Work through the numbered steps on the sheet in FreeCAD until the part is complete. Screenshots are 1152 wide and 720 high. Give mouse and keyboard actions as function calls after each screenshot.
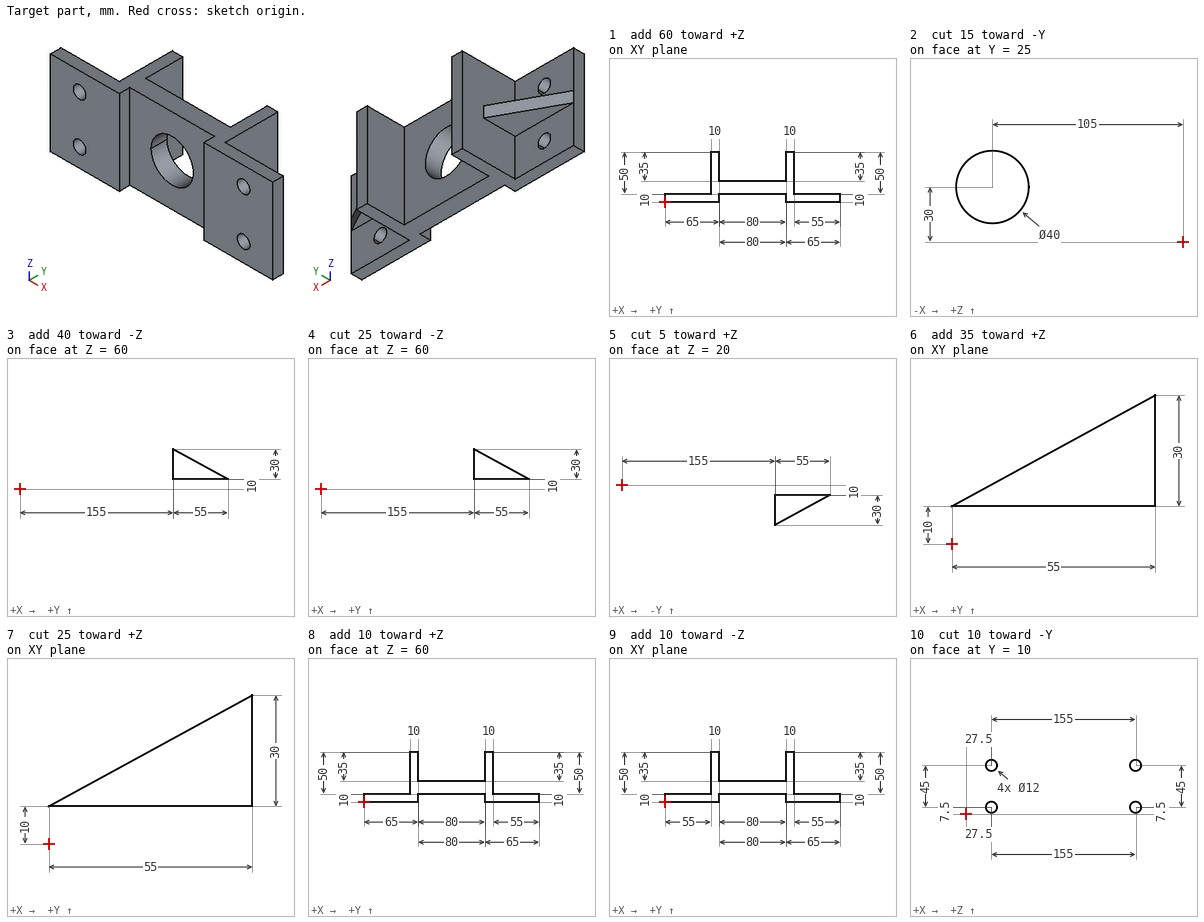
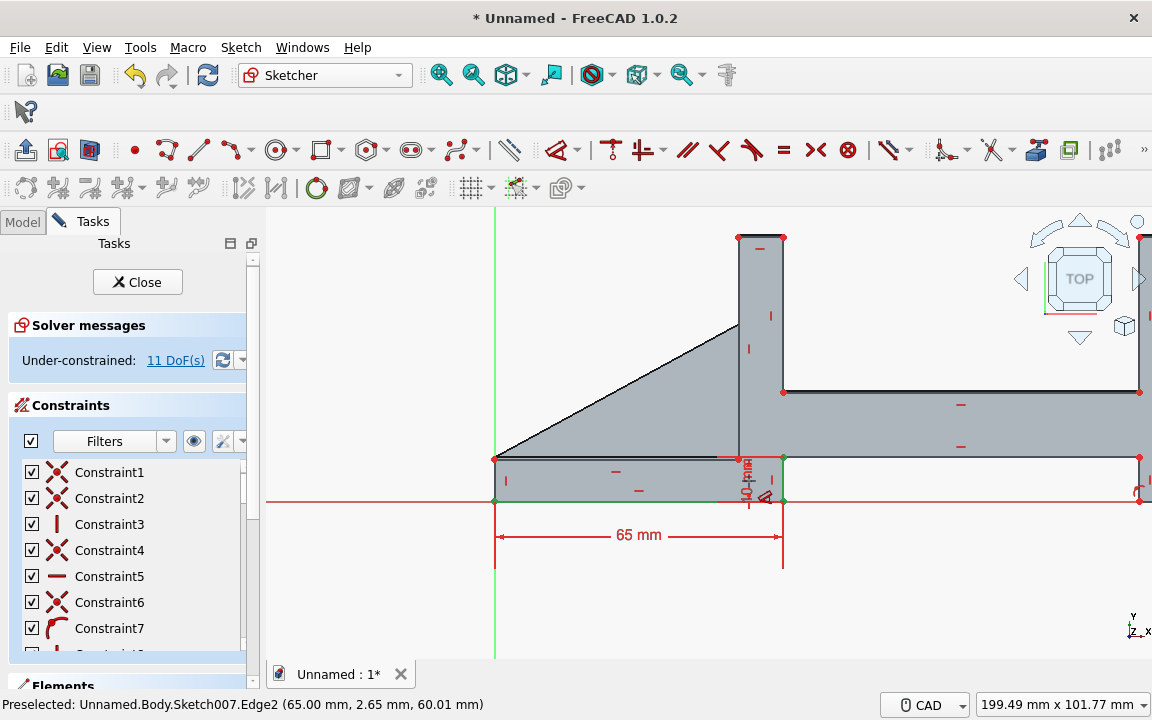
click(890, 457)
click(885, 423)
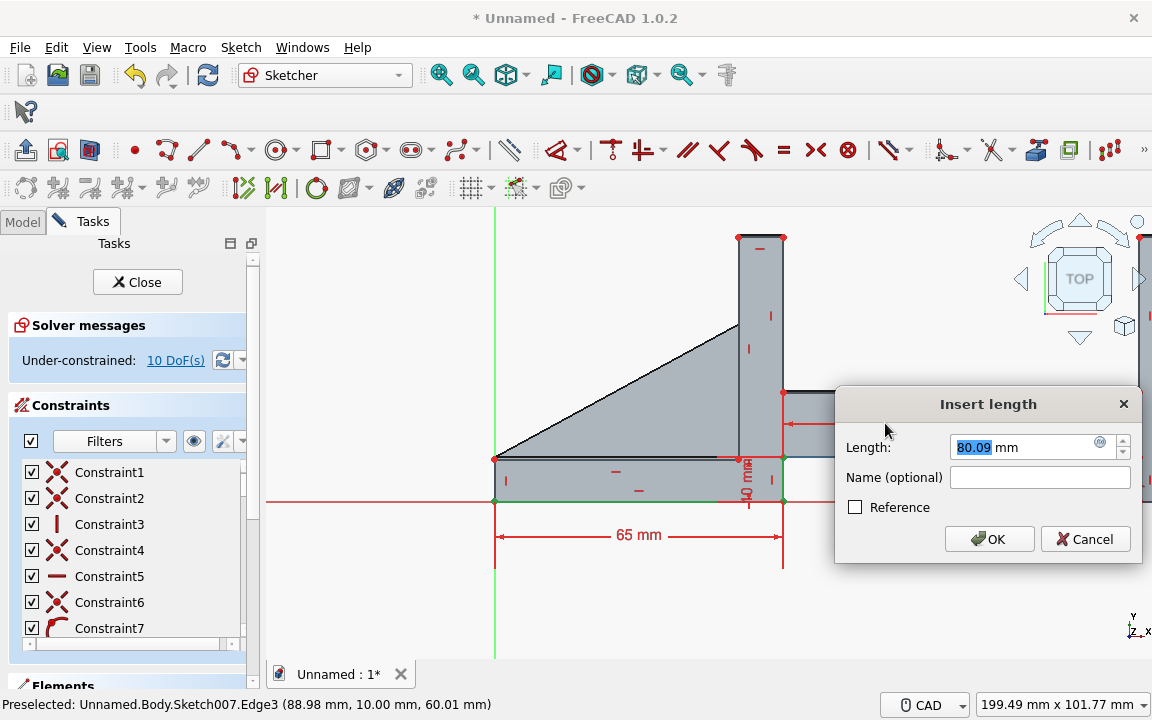
text(80)
key(Return)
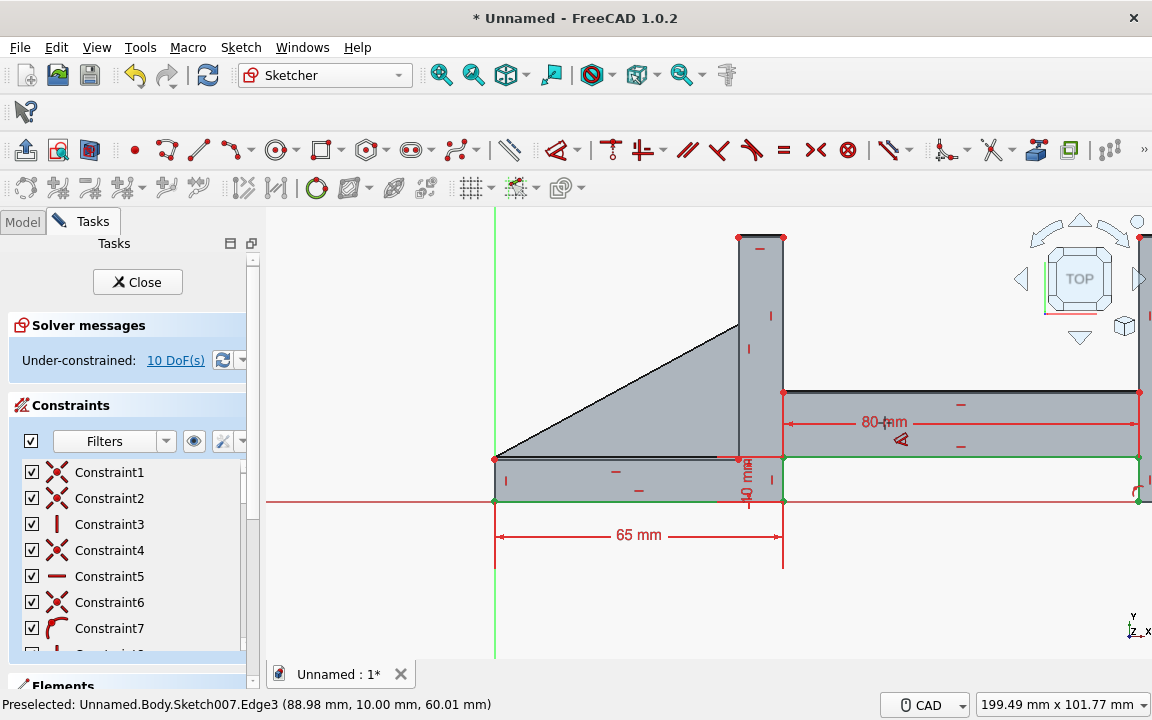
scroll(294, 511, down, 3)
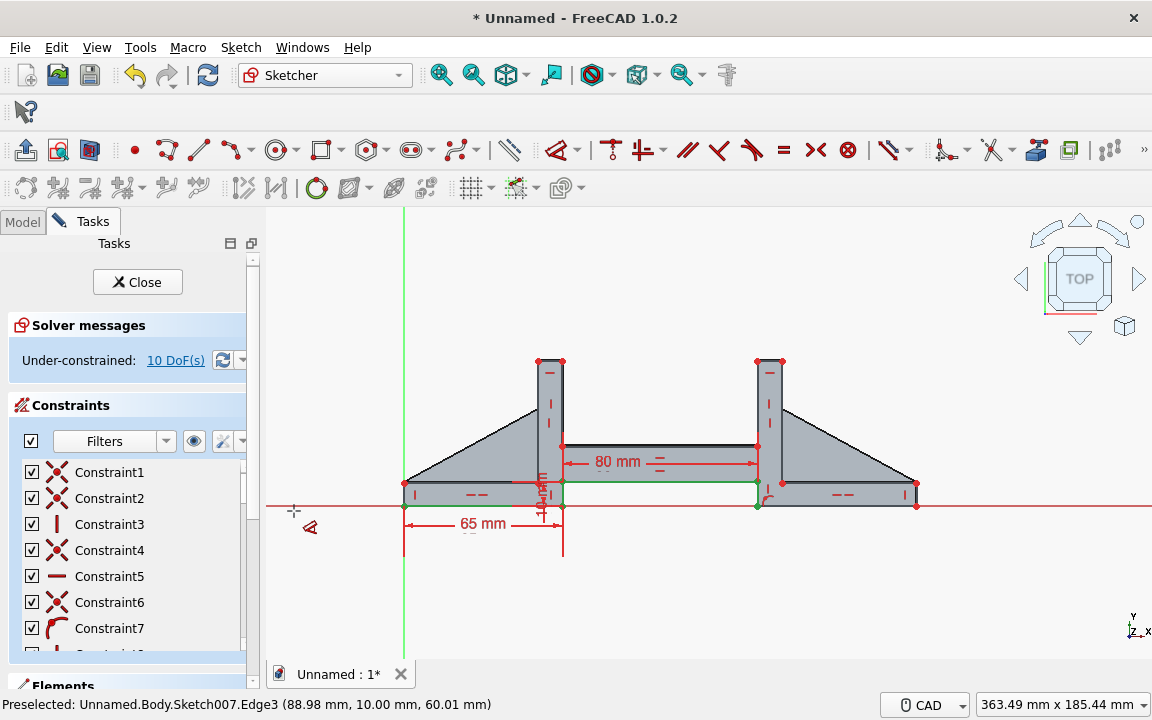
click(805, 506)
click(837, 540)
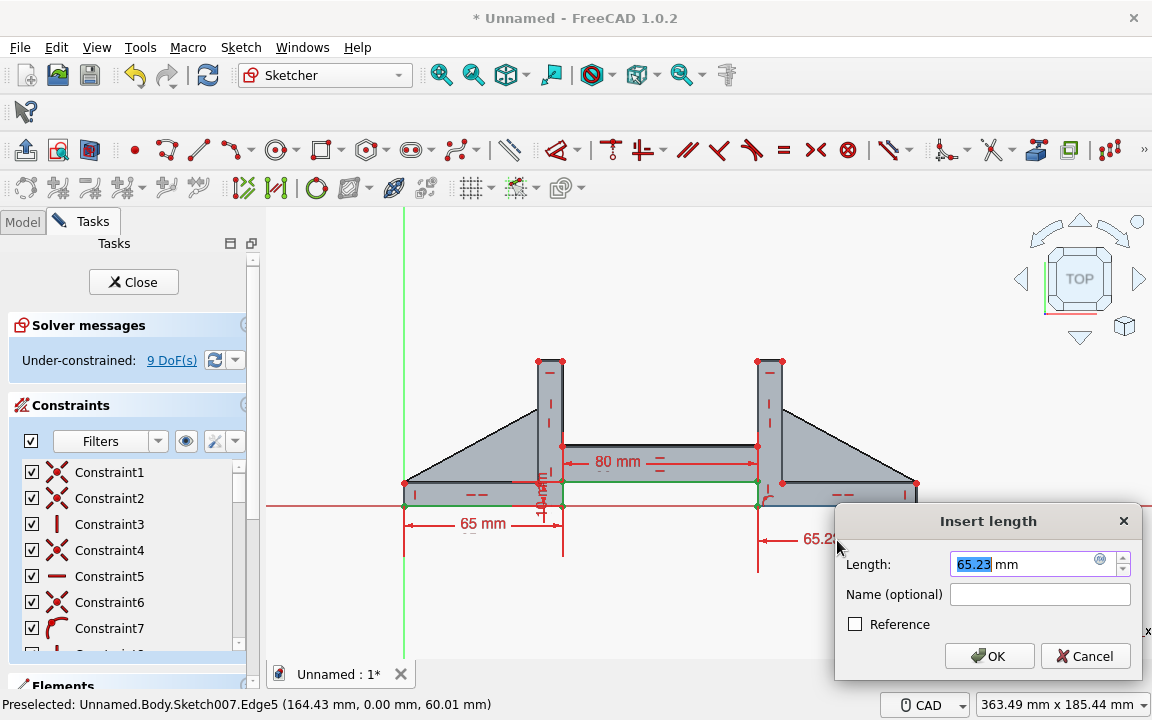
text(65)
key(Return)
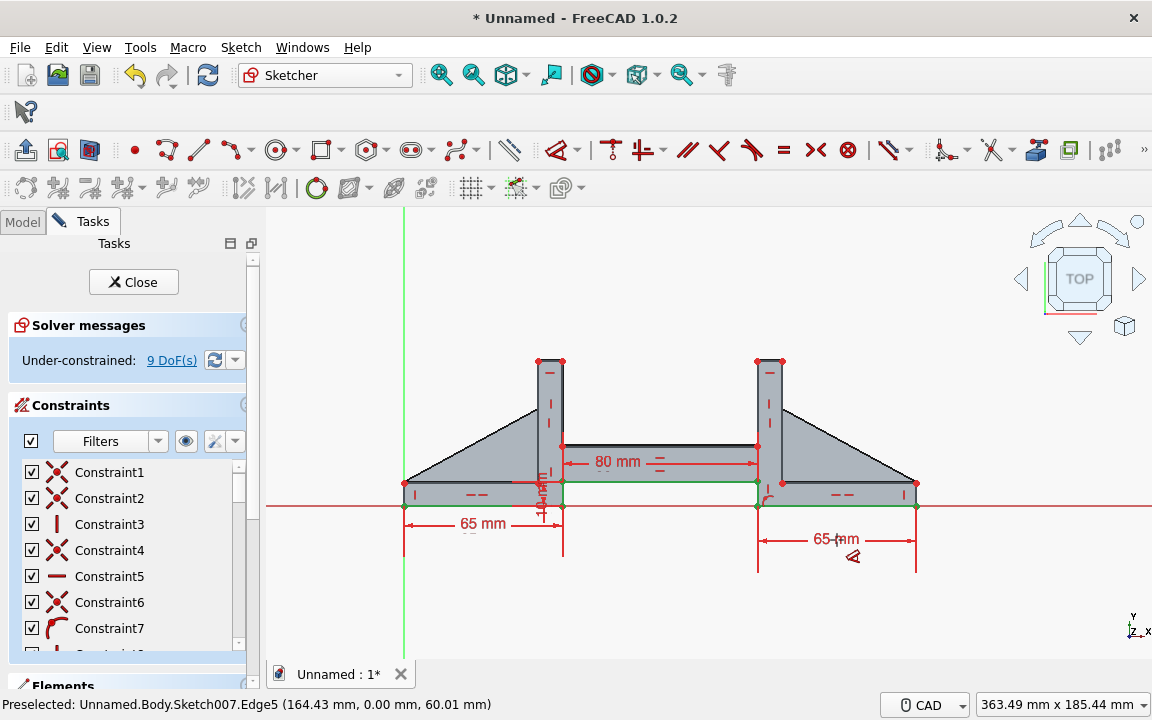
scroll(916, 497, up, 3)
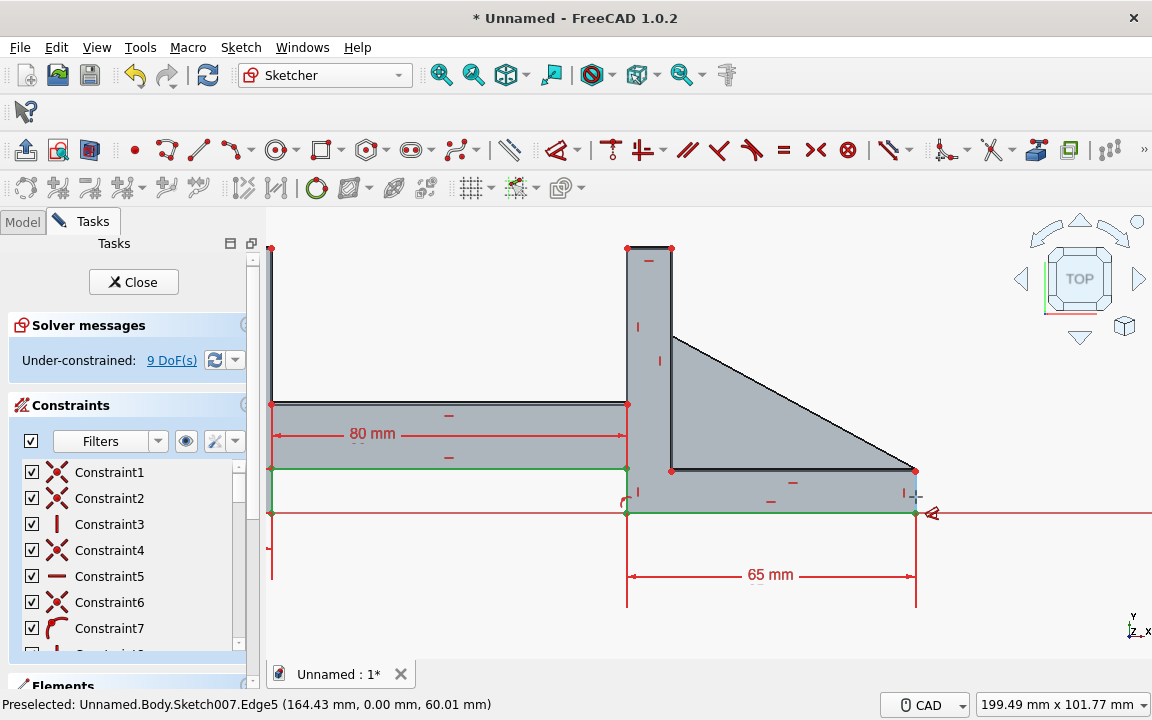
click(916, 496)
click(950, 492)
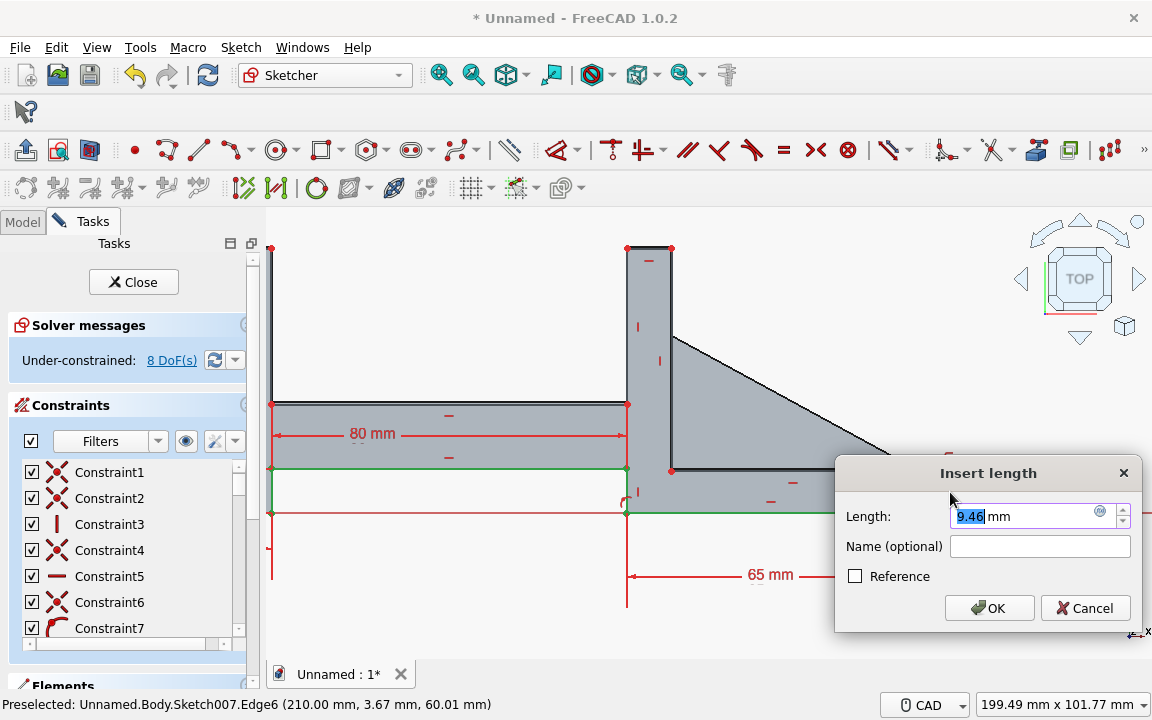
text(10)
key(Return)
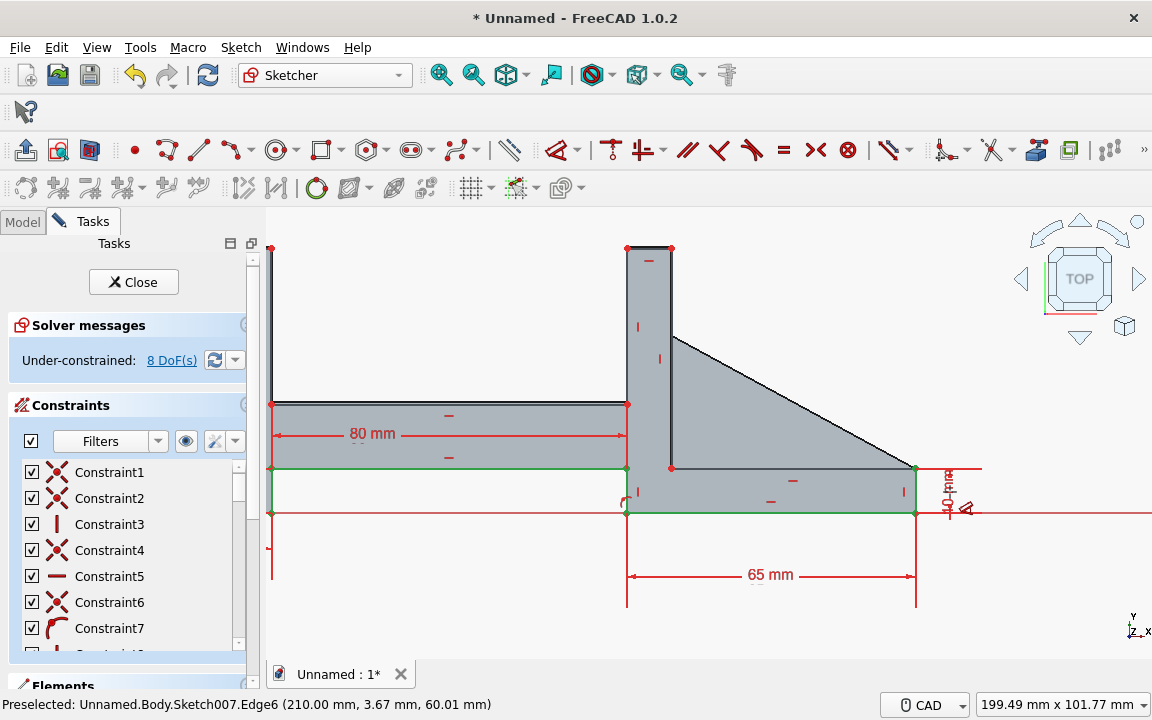
click(842, 469)
click(794, 435)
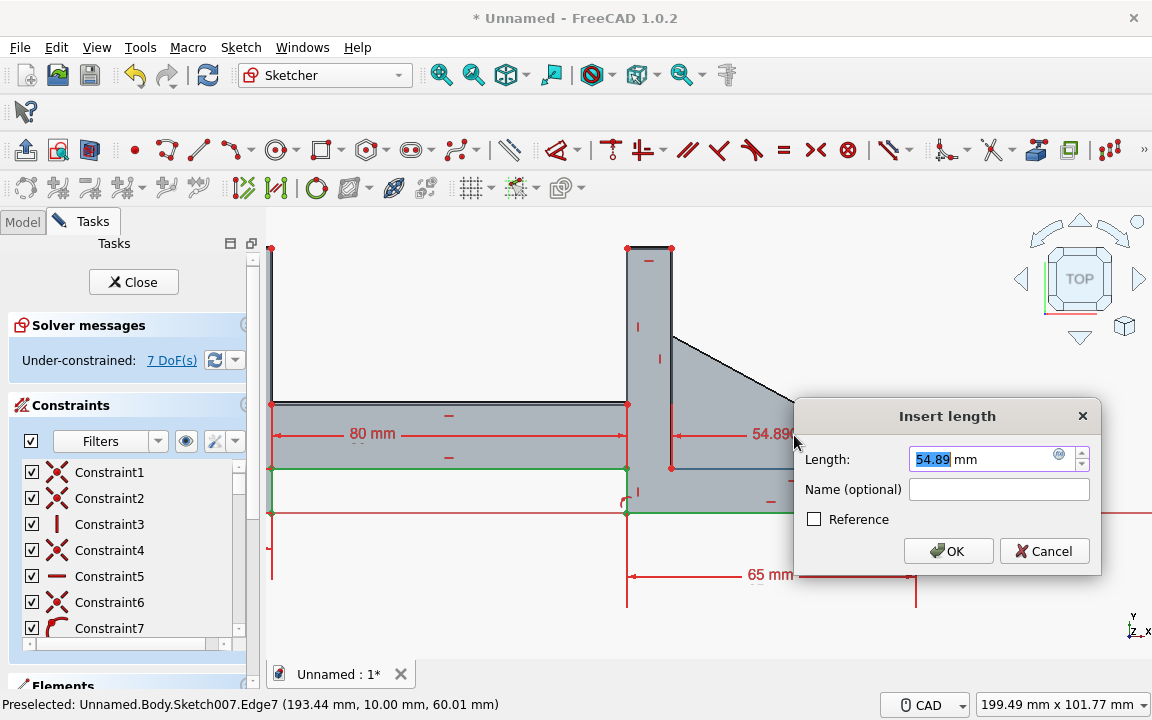
text(55)
key(Return)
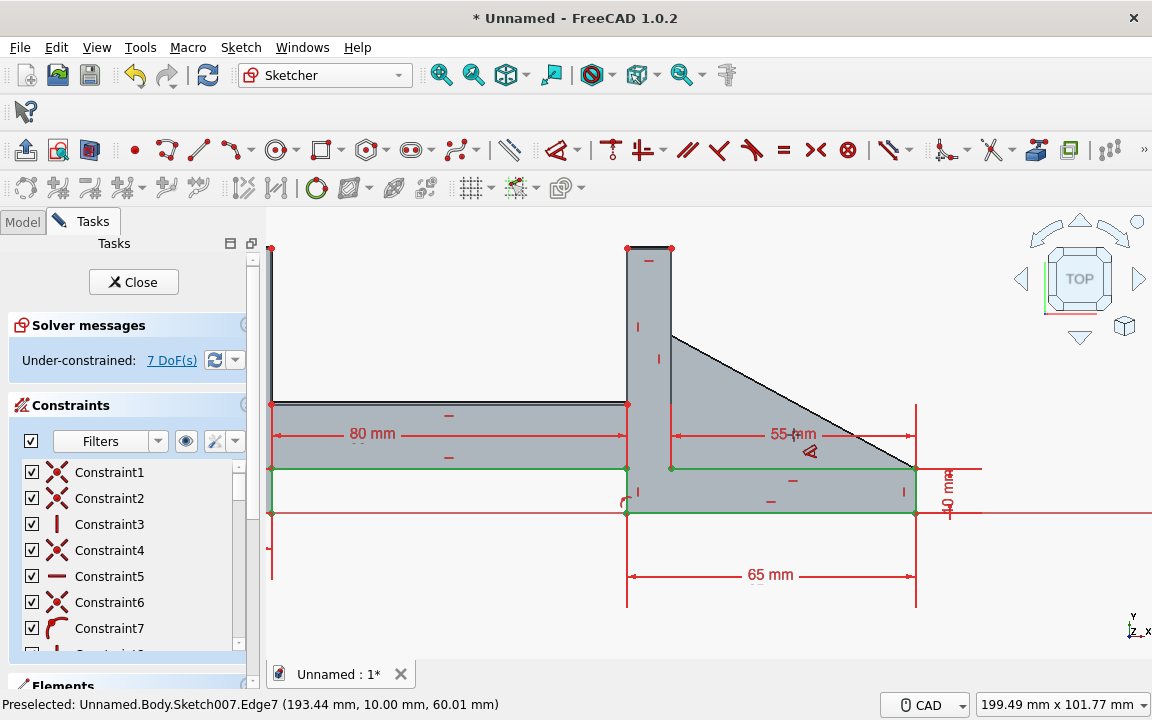
click(671, 403)
click(705, 359)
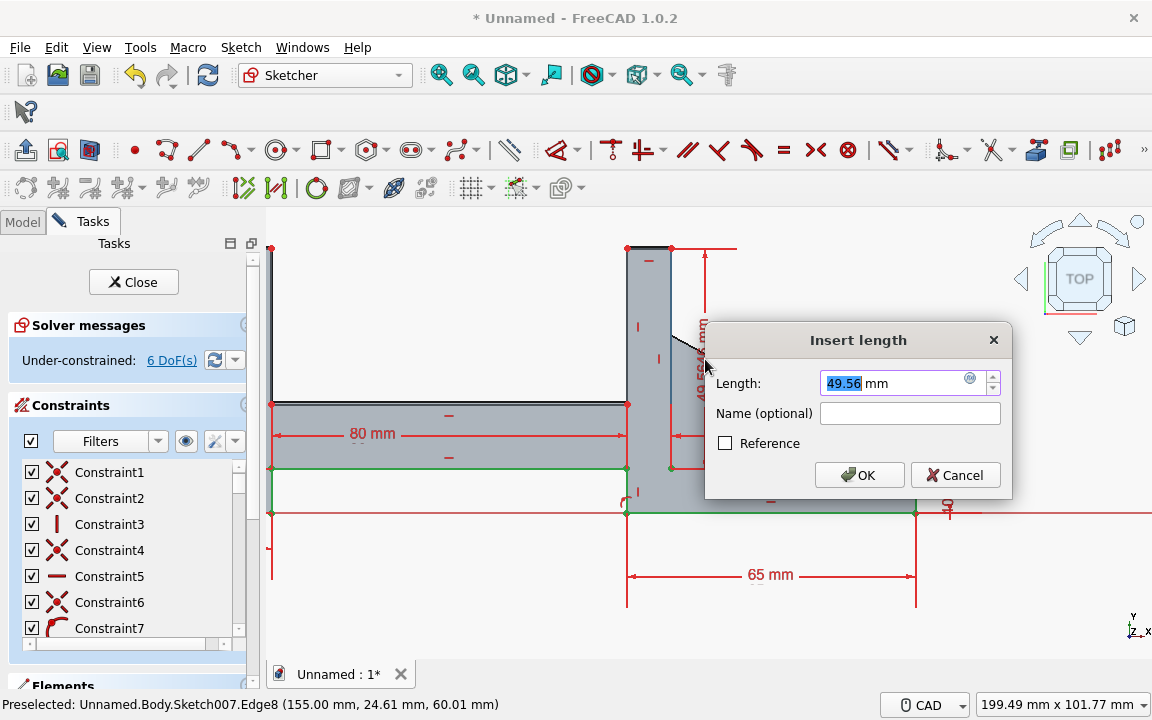
text(50)
key(Return)